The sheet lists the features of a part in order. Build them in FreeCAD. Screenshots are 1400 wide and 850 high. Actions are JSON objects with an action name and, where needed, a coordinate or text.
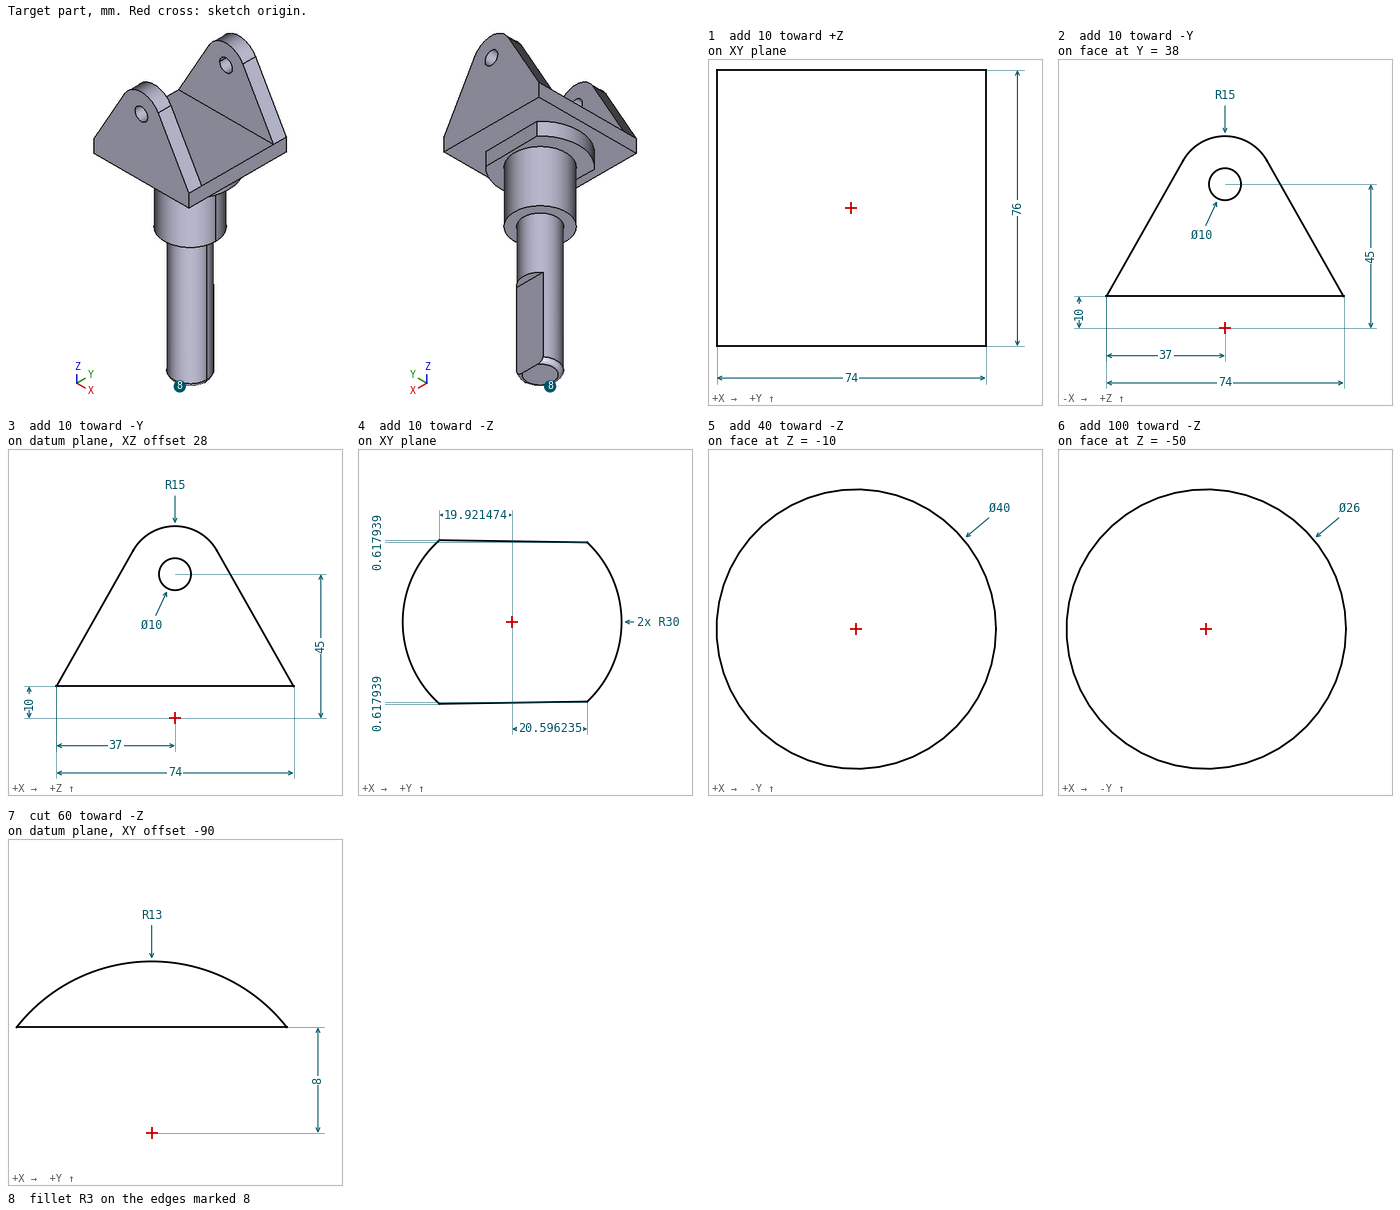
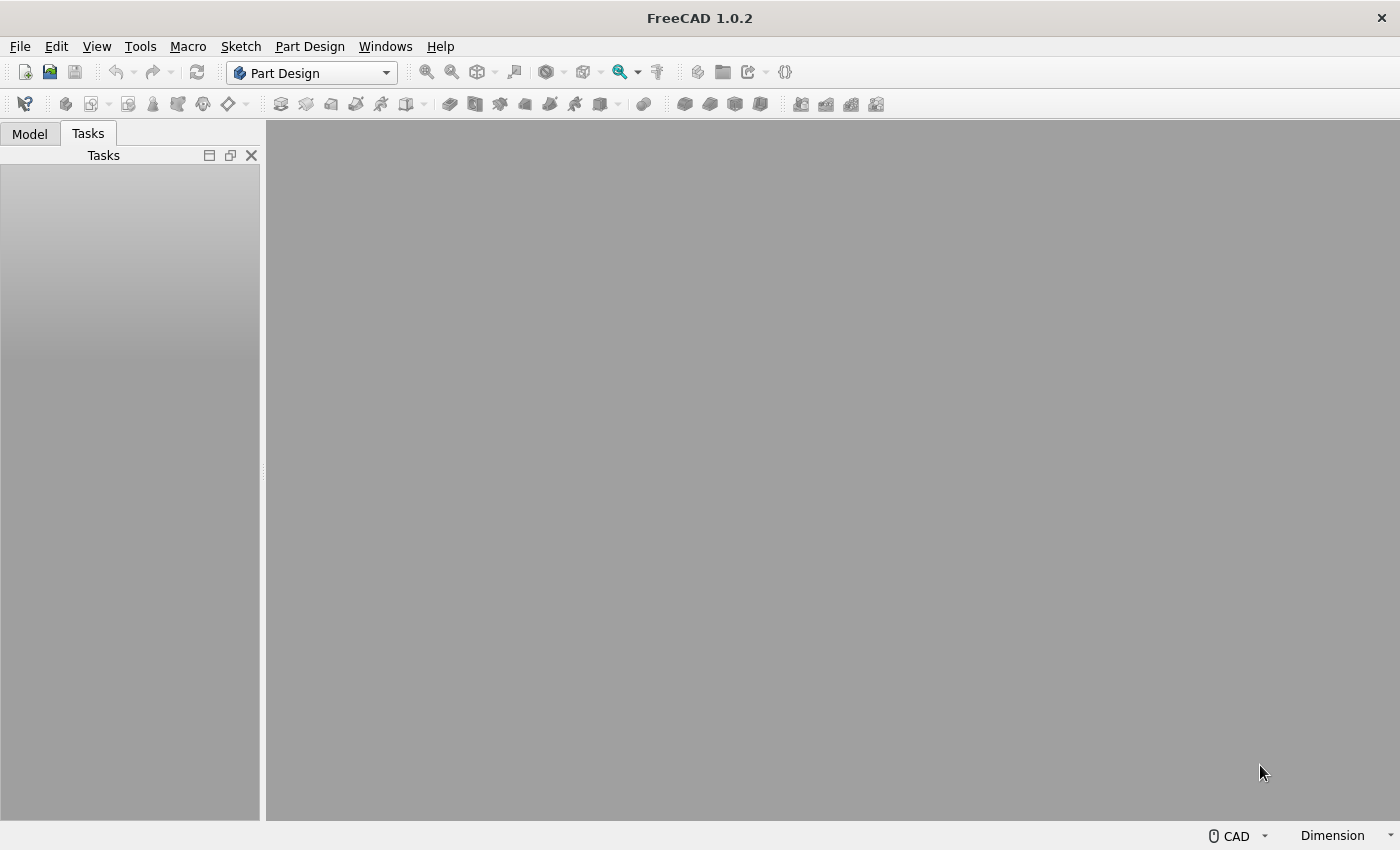
{"action": "left_click", "coordinate": [25, 72]}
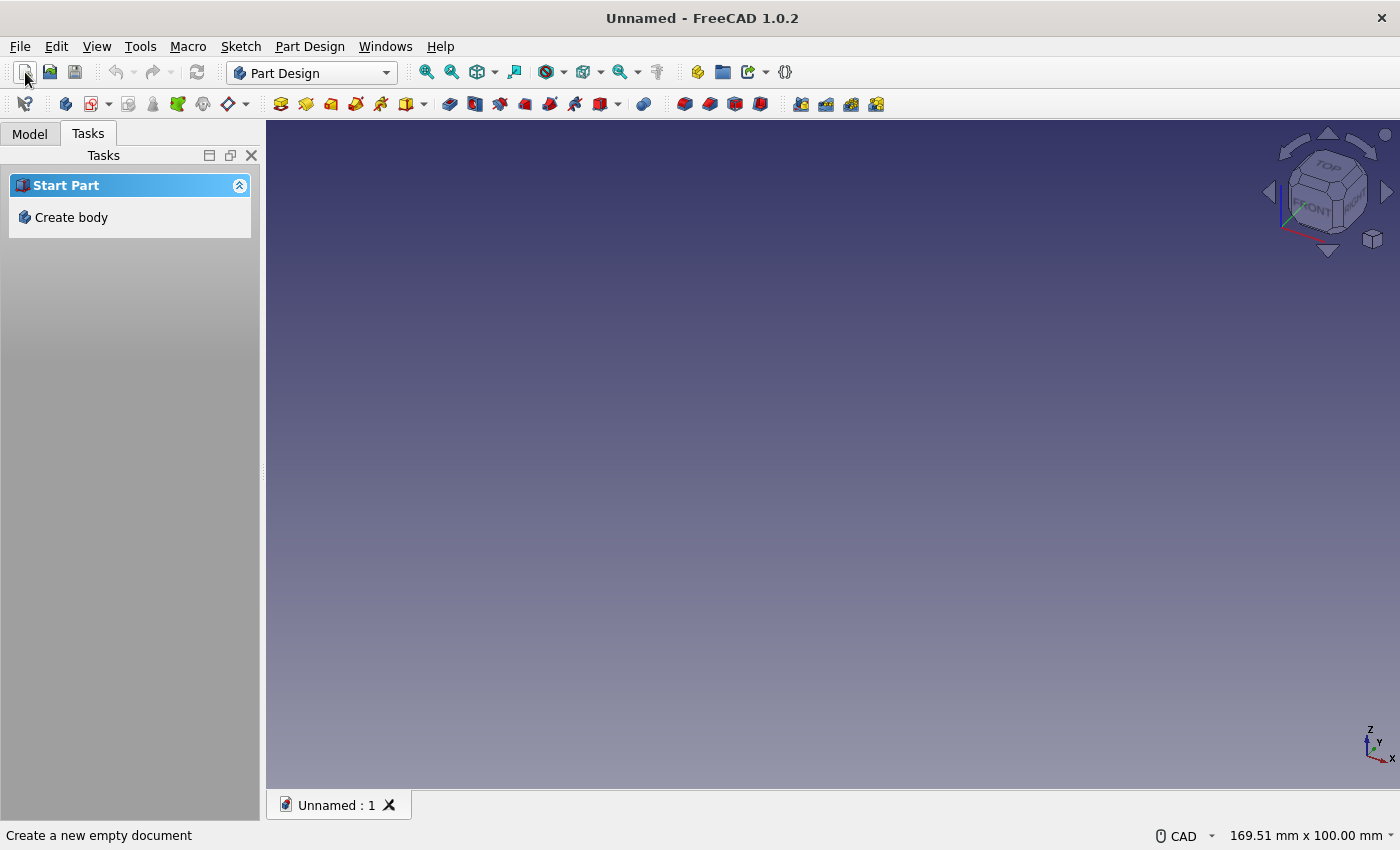
{"action": "left_click", "coordinate": [90, 104]}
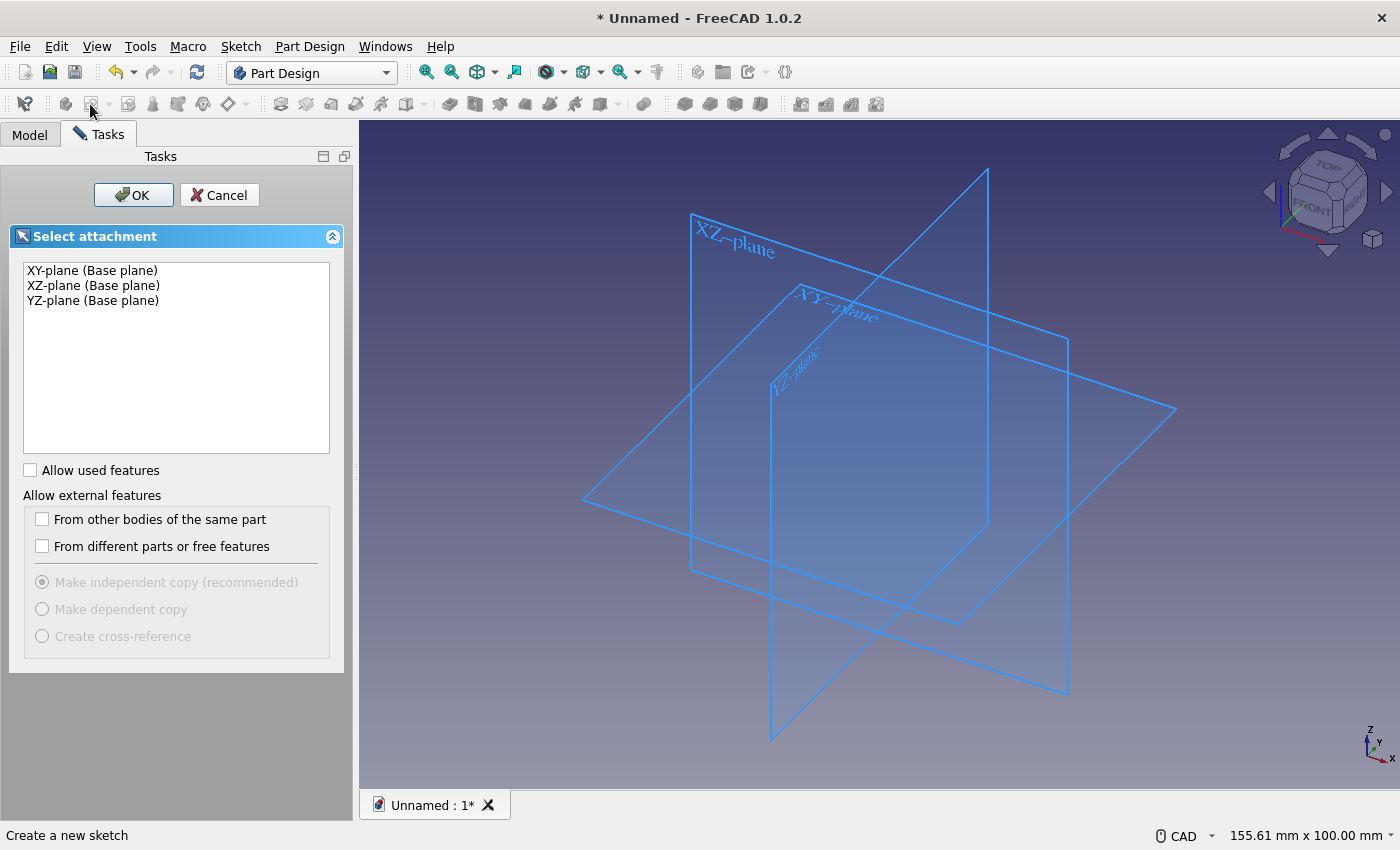
{"action": "left_click", "coordinate": [84, 270]}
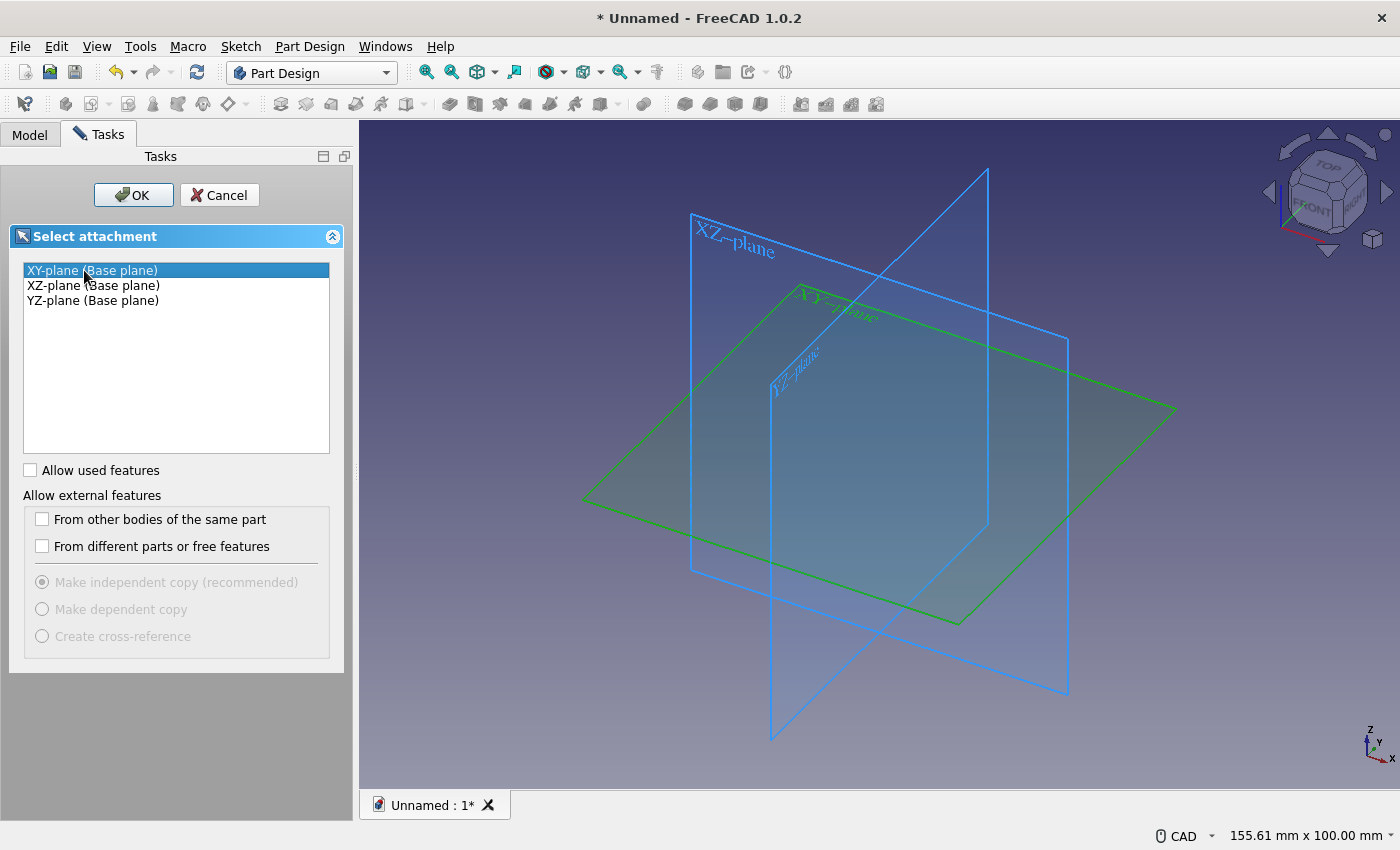
{"action": "left_click", "coordinate": [134, 195]}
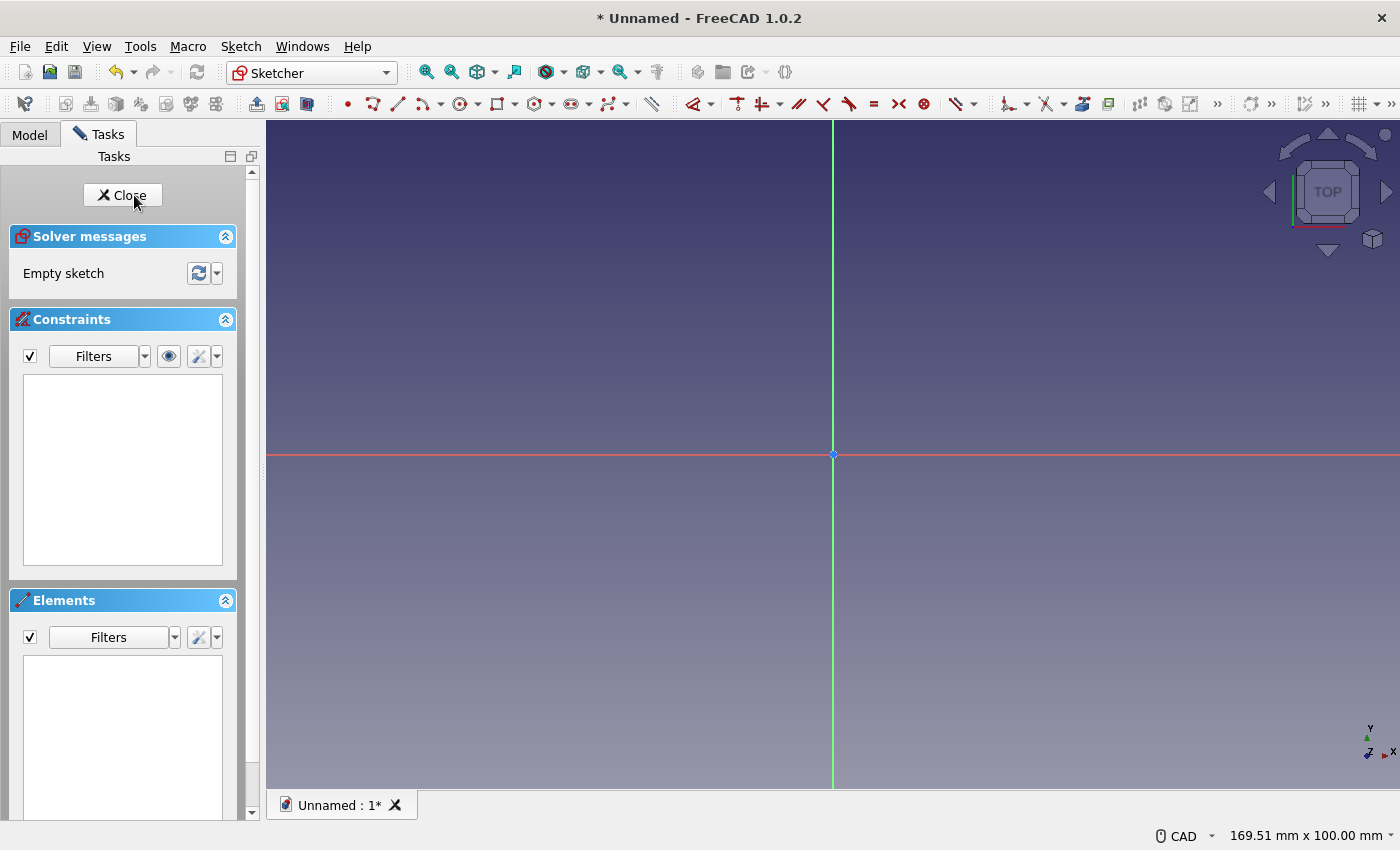
{"action": "left_click", "coordinate": [514, 104]}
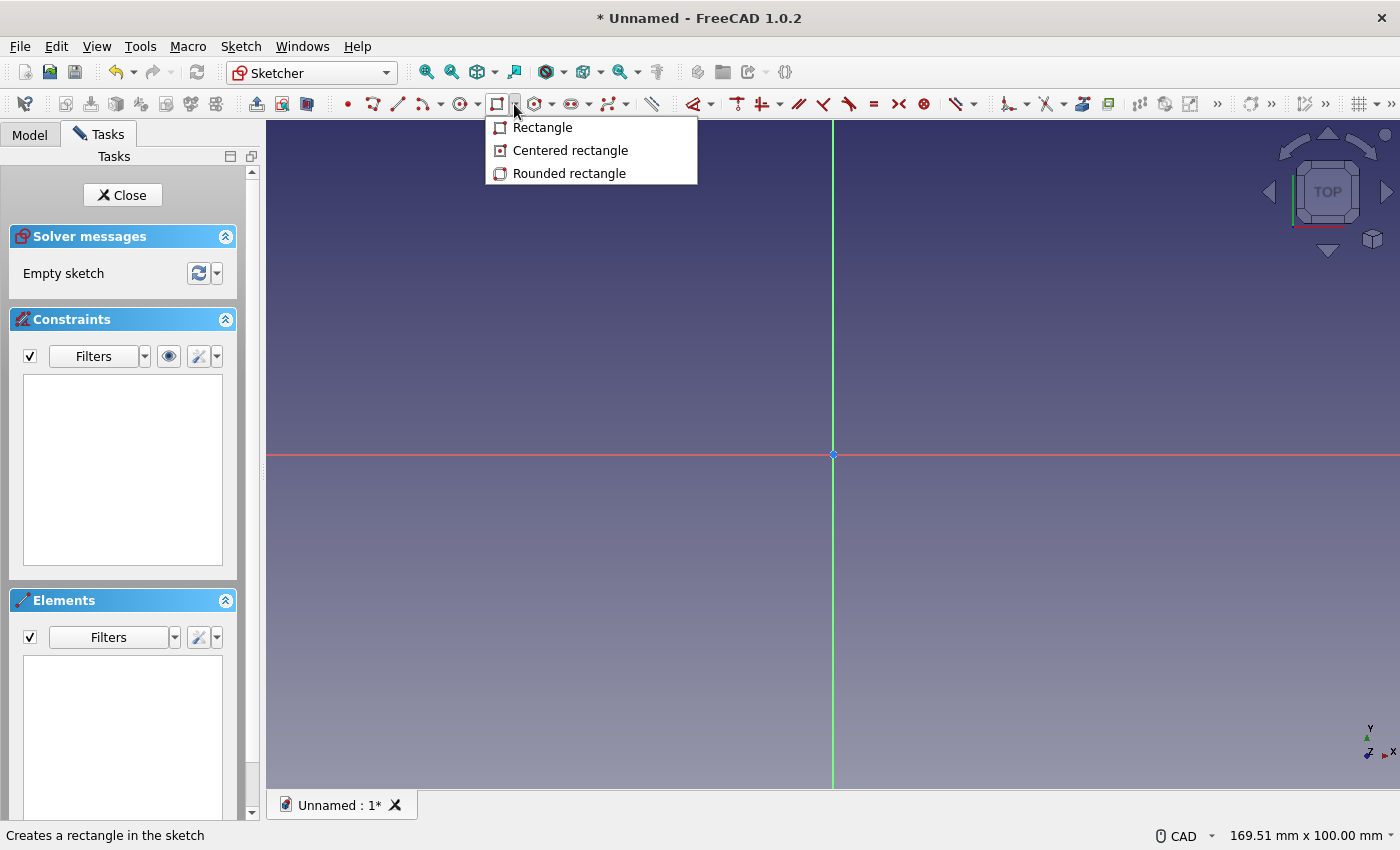
{"action": "left_click", "coordinate": [592, 150]}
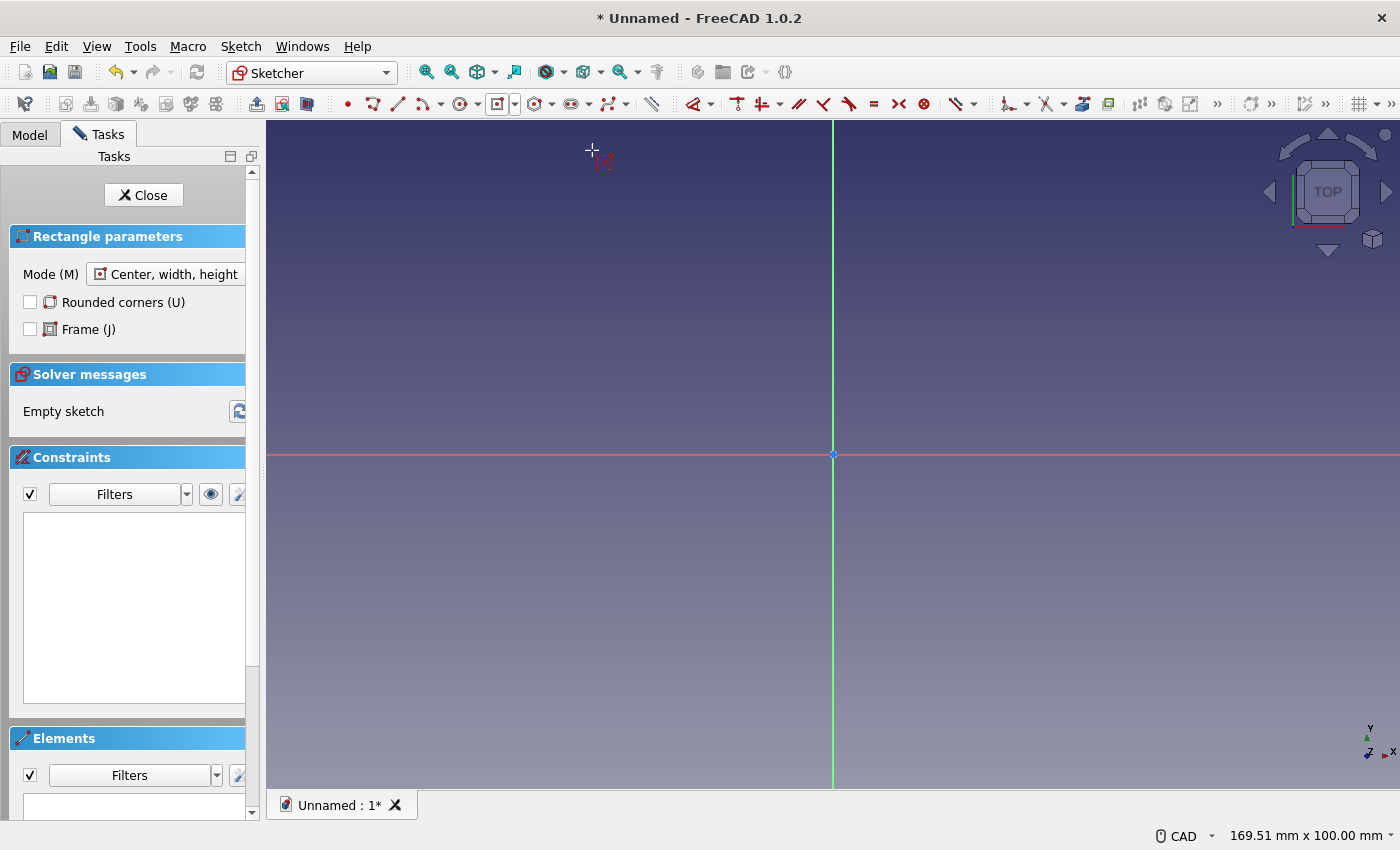
{"action": "left_click", "coordinate": [833, 454]}
{"action": "left_click", "coordinate": [1081, 200]}
{"action": "key", "text": "Escape"}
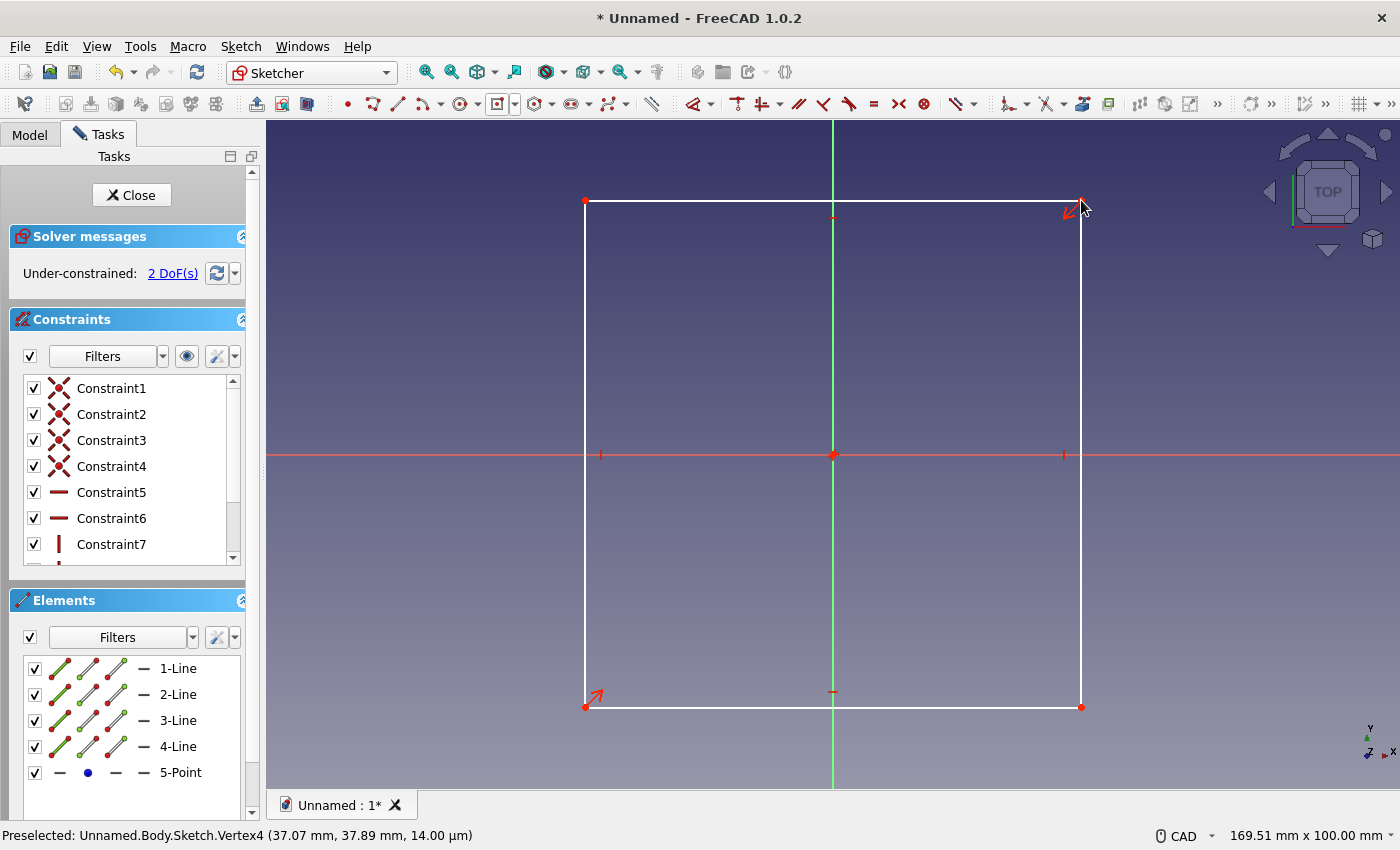
{"action": "left_click", "coordinate": [734, 708]}